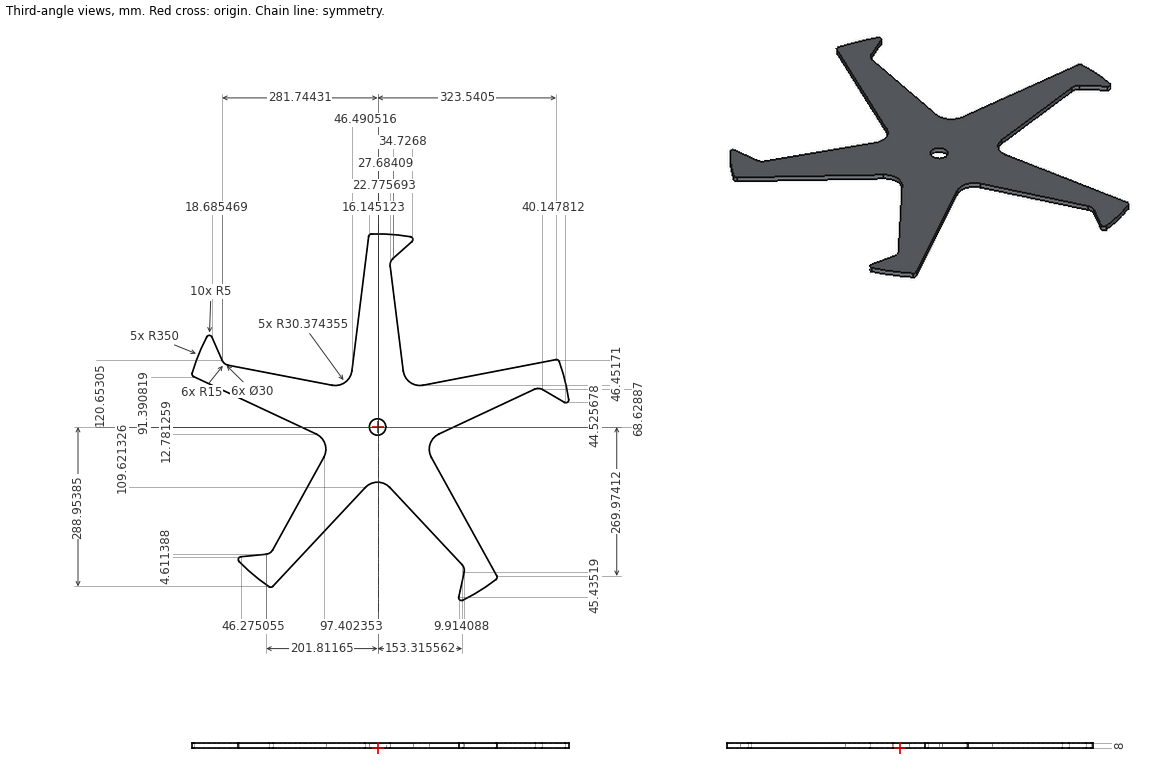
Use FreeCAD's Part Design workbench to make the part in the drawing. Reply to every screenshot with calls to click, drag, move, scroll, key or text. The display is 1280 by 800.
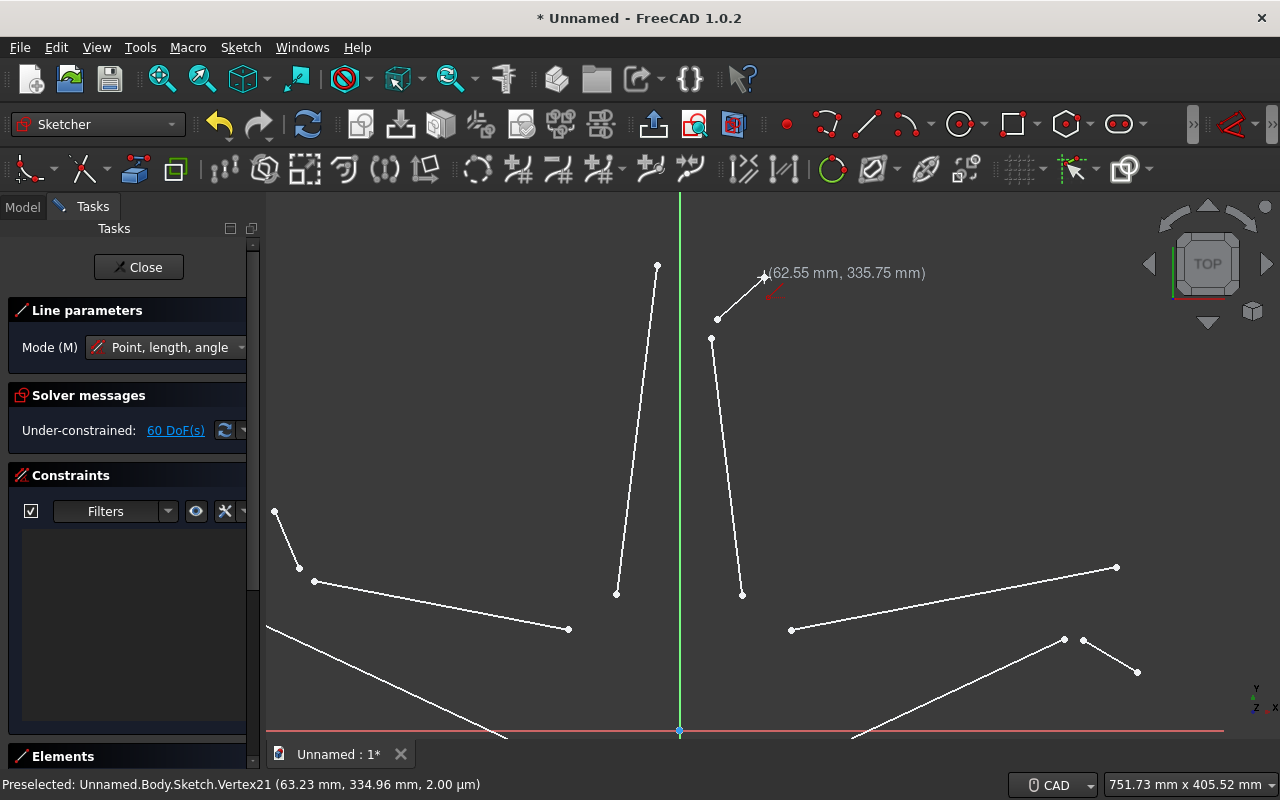
click(934, 124)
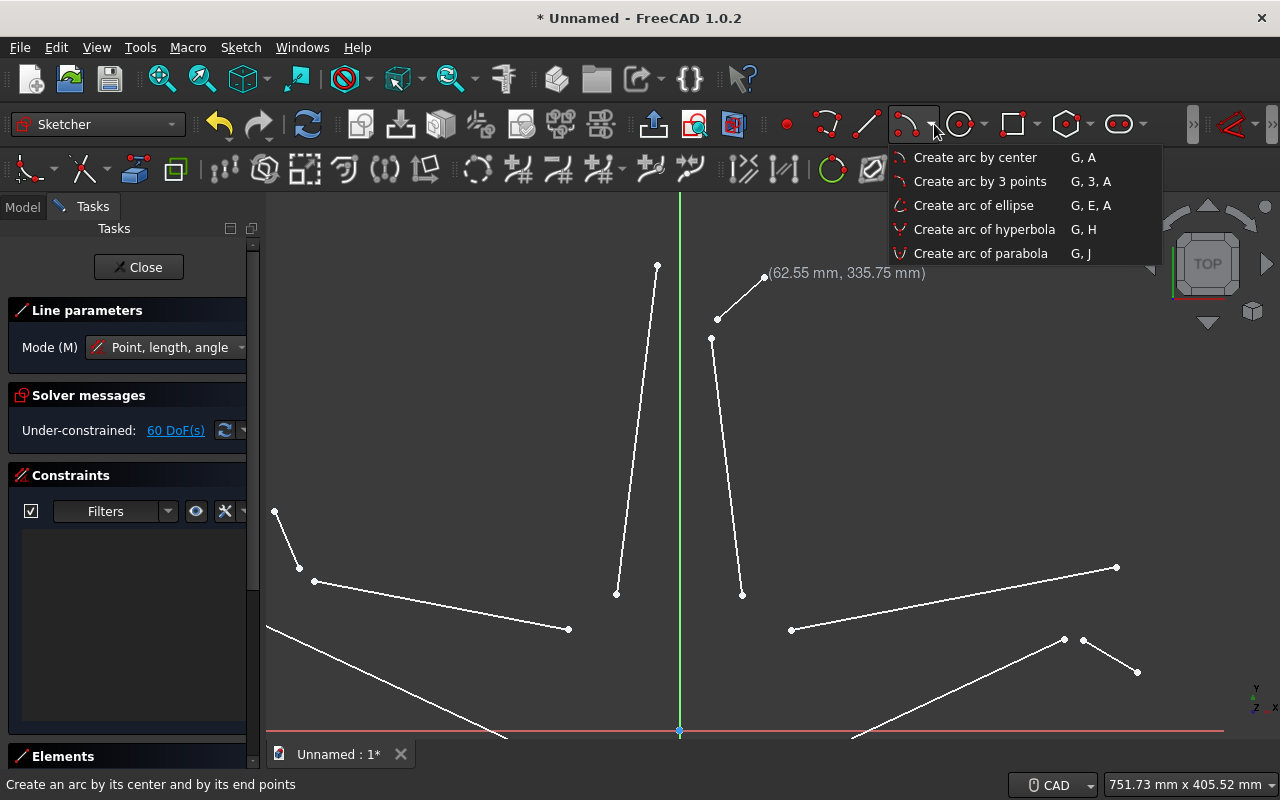
click(1026, 181)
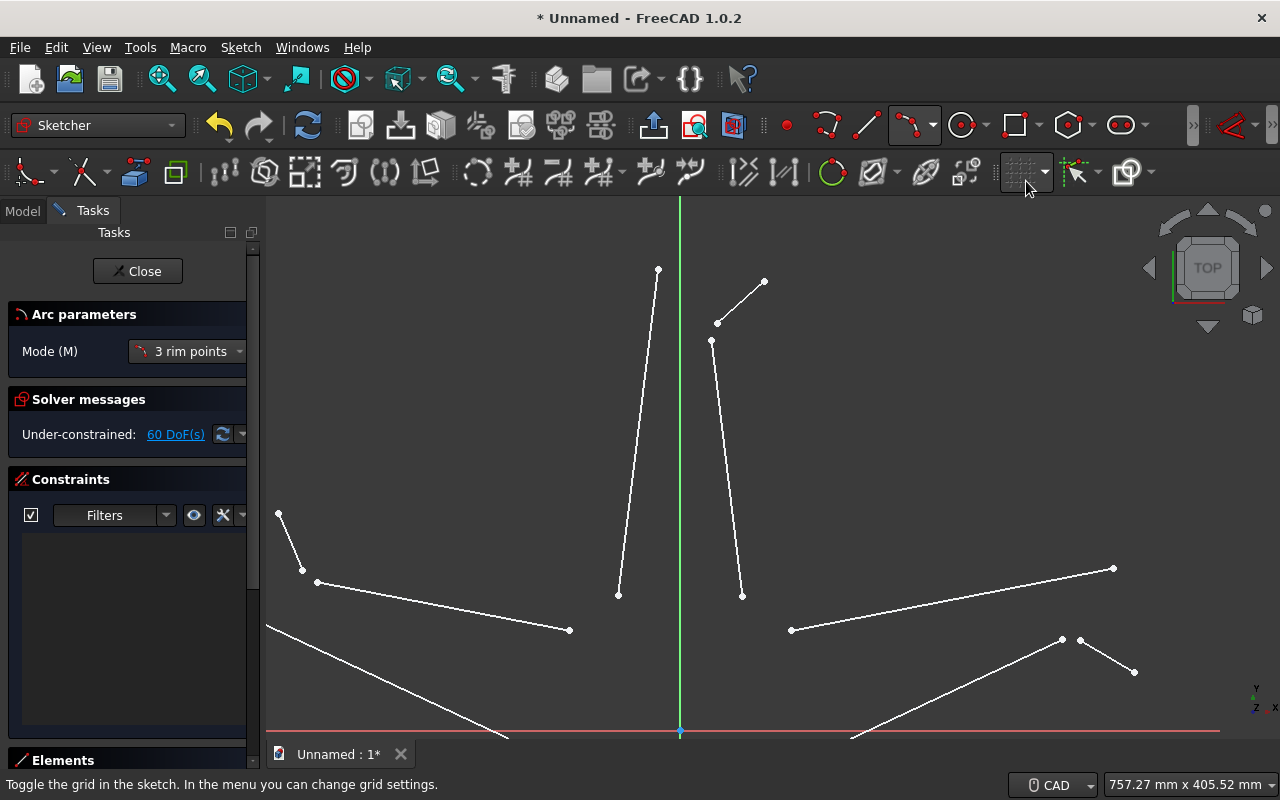
click(618, 596)
click(570, 631)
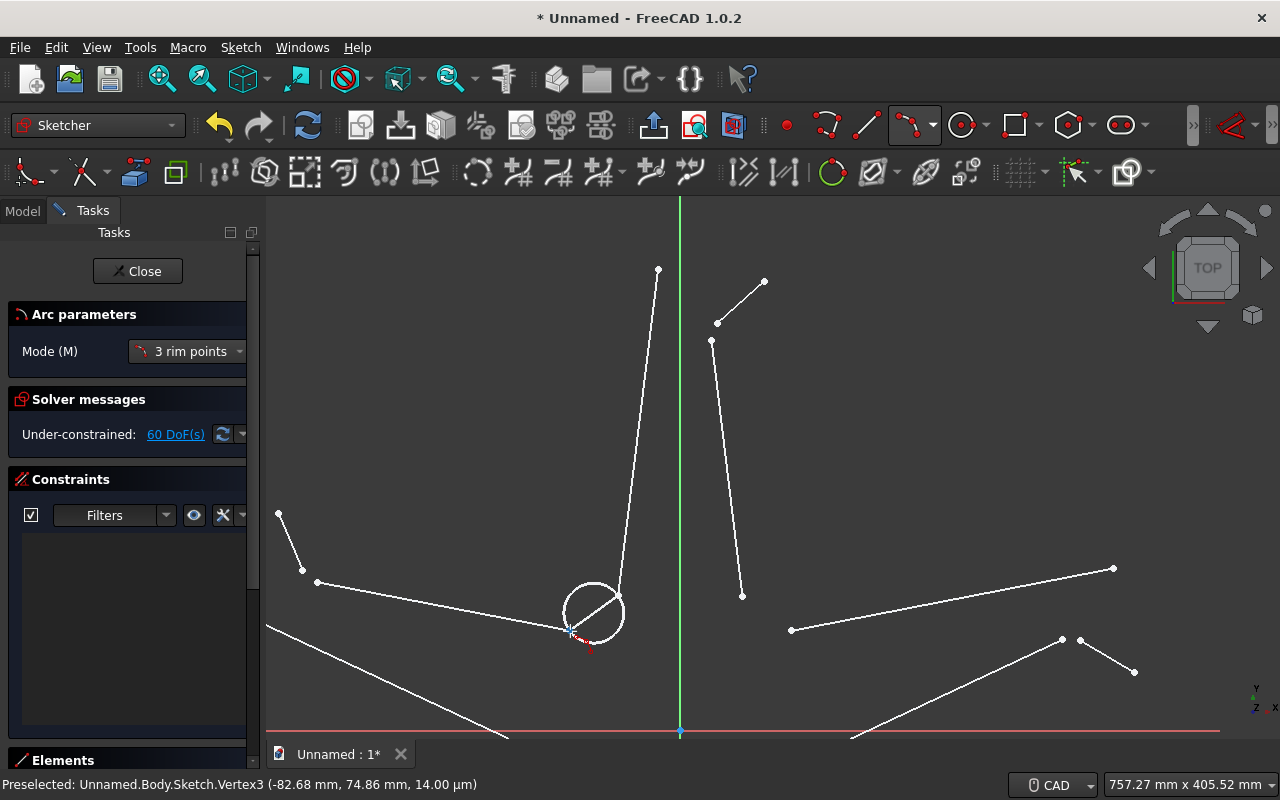
scroll(602, 623, up, 2)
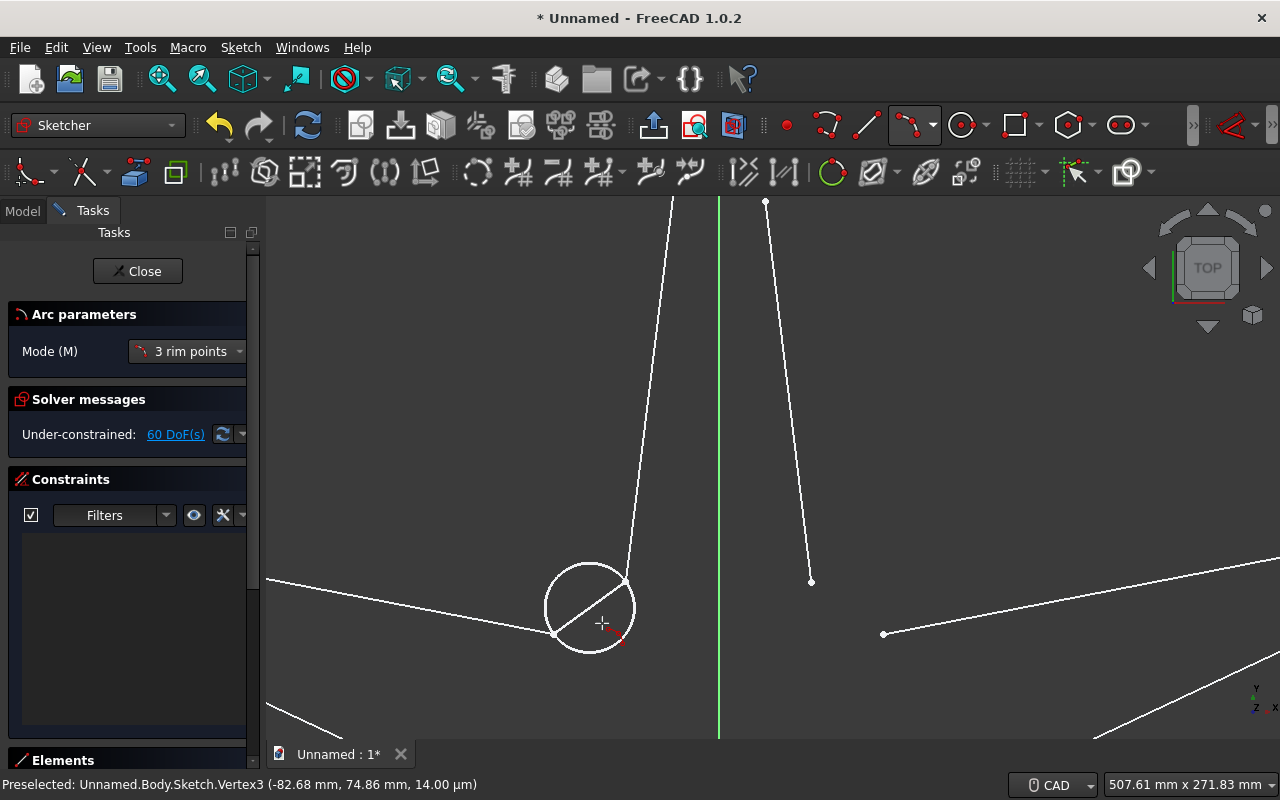
click(601, 622)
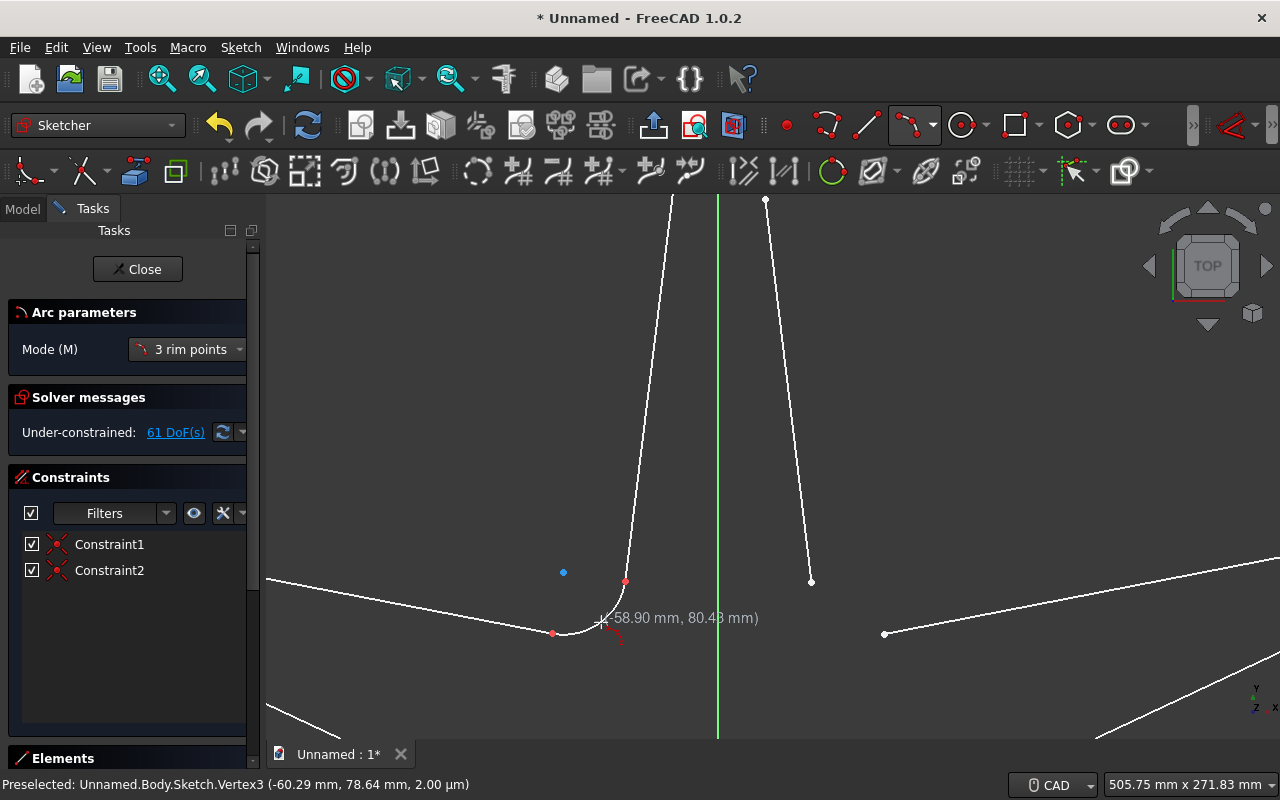
scroll(697, 374, down, 7)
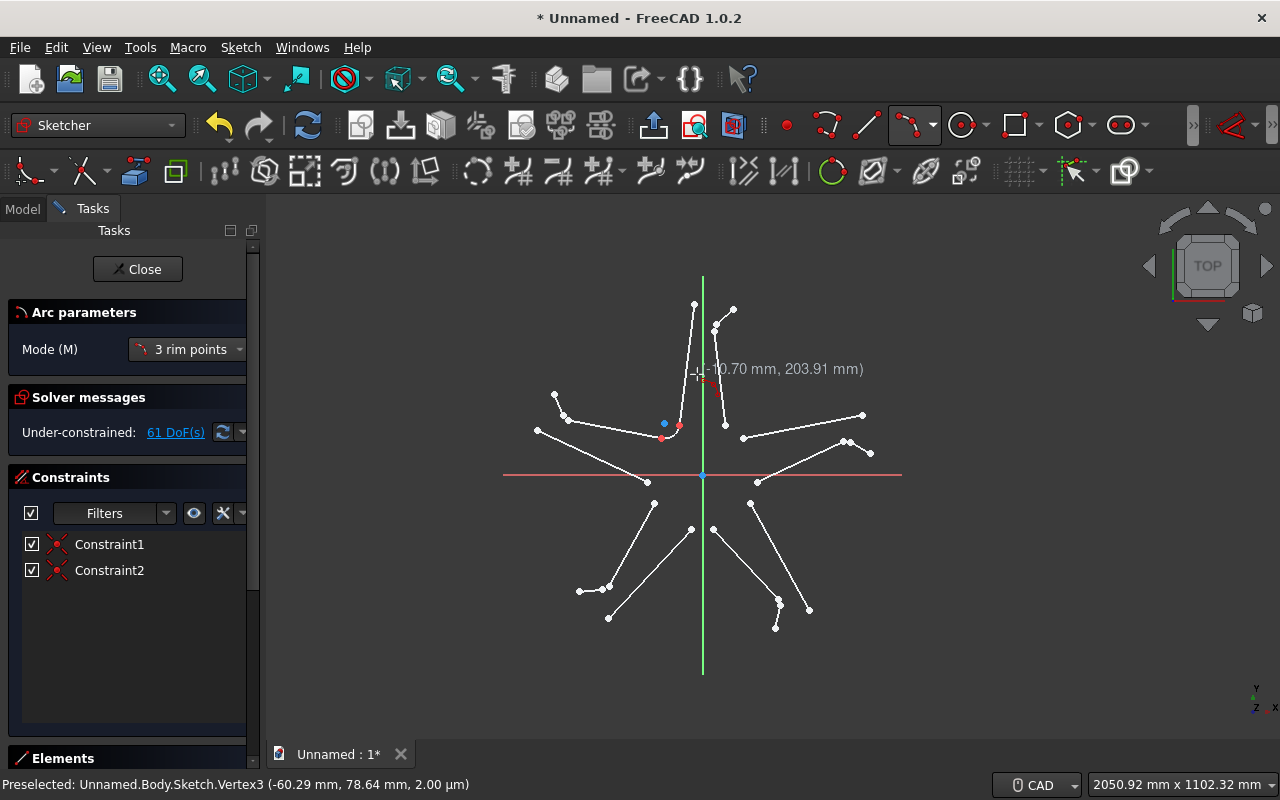
scroll(569, 420, up, 5)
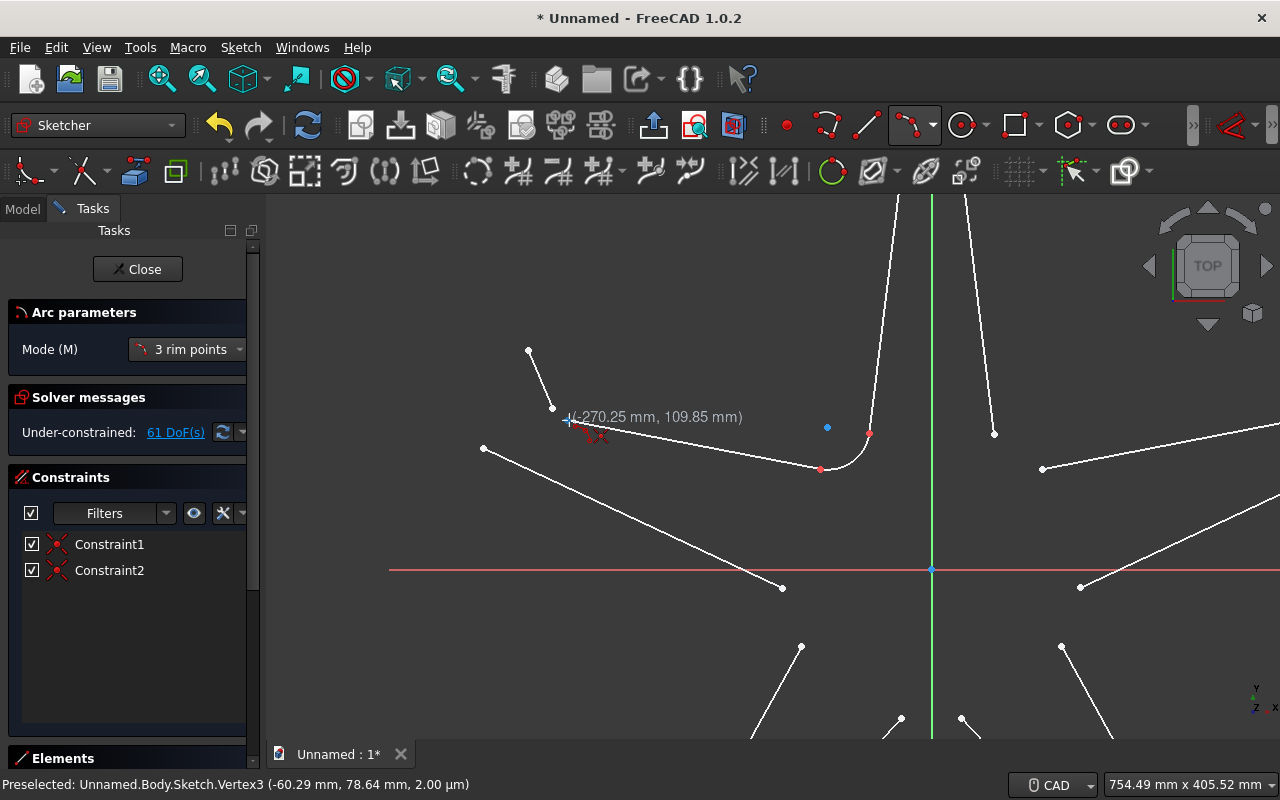
click(567, 420)
click(553, 408)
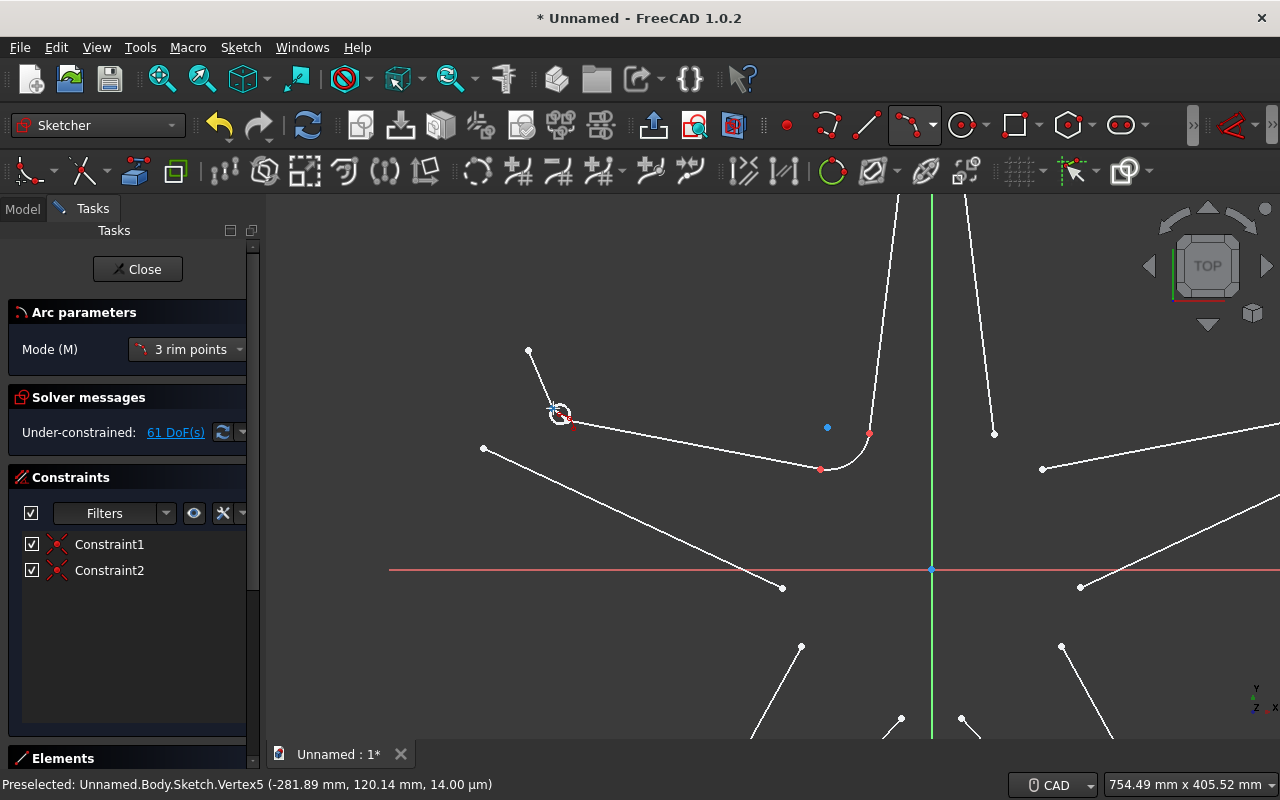
scroll(559, 415, up, 10)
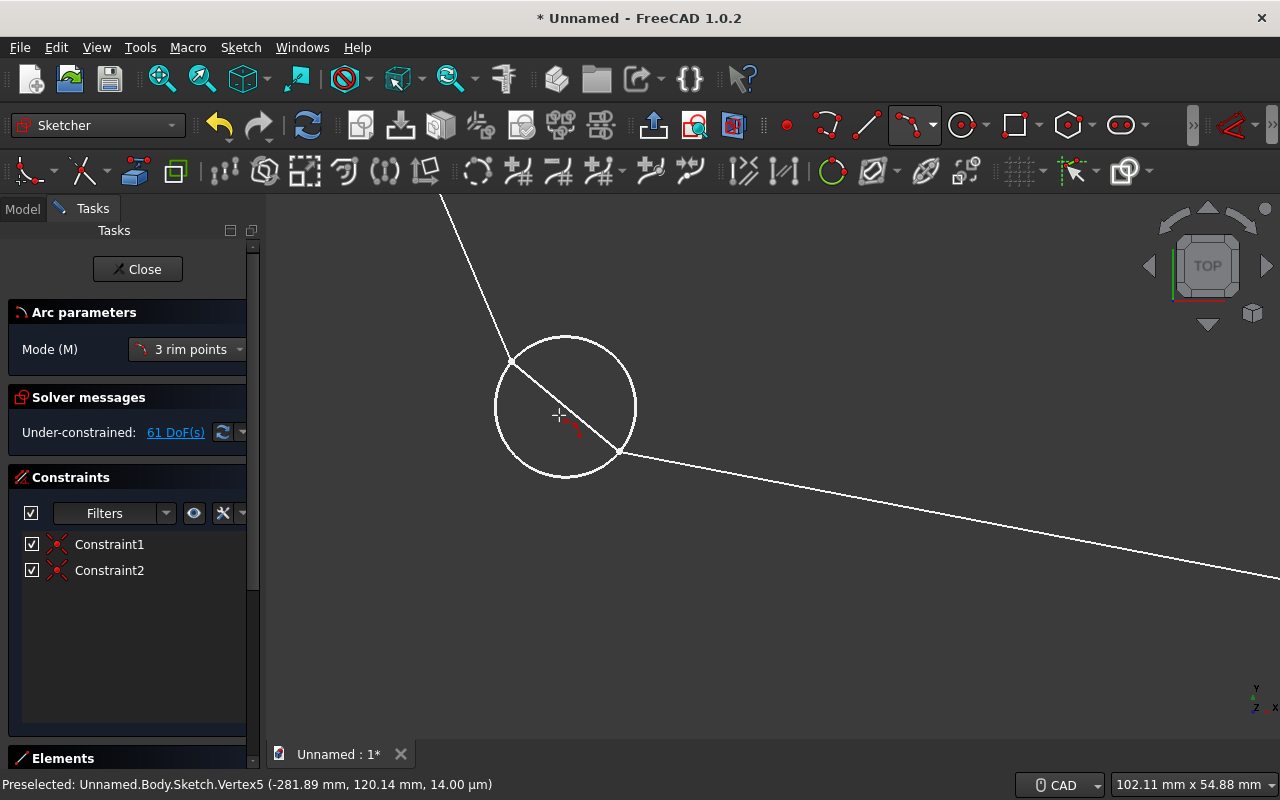
click(557, 413)